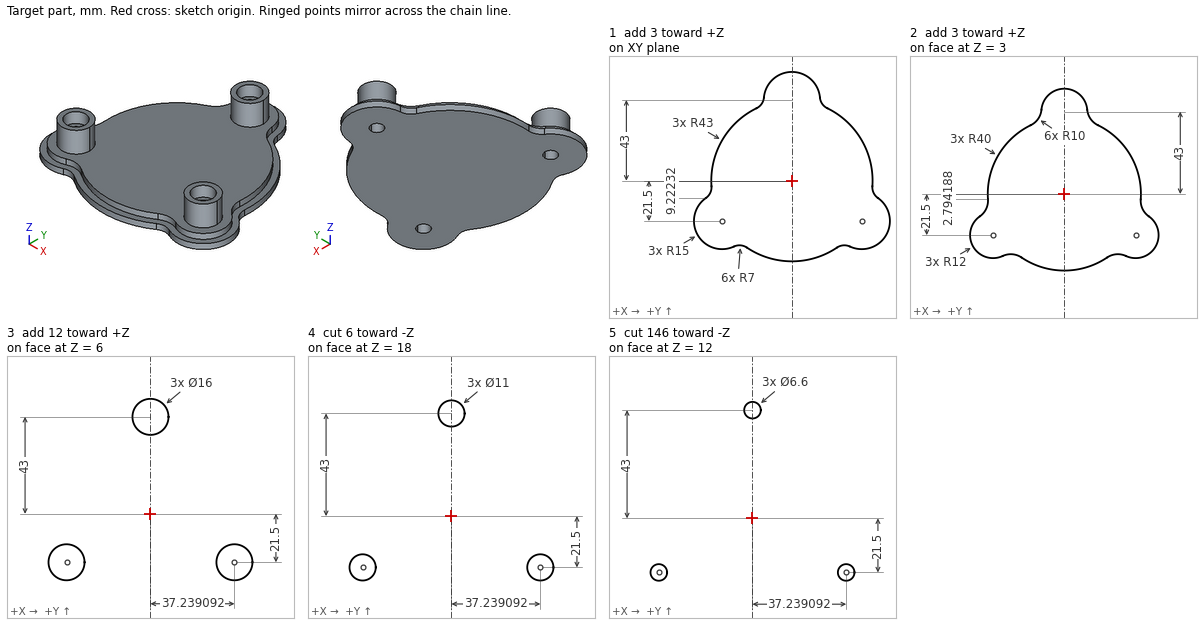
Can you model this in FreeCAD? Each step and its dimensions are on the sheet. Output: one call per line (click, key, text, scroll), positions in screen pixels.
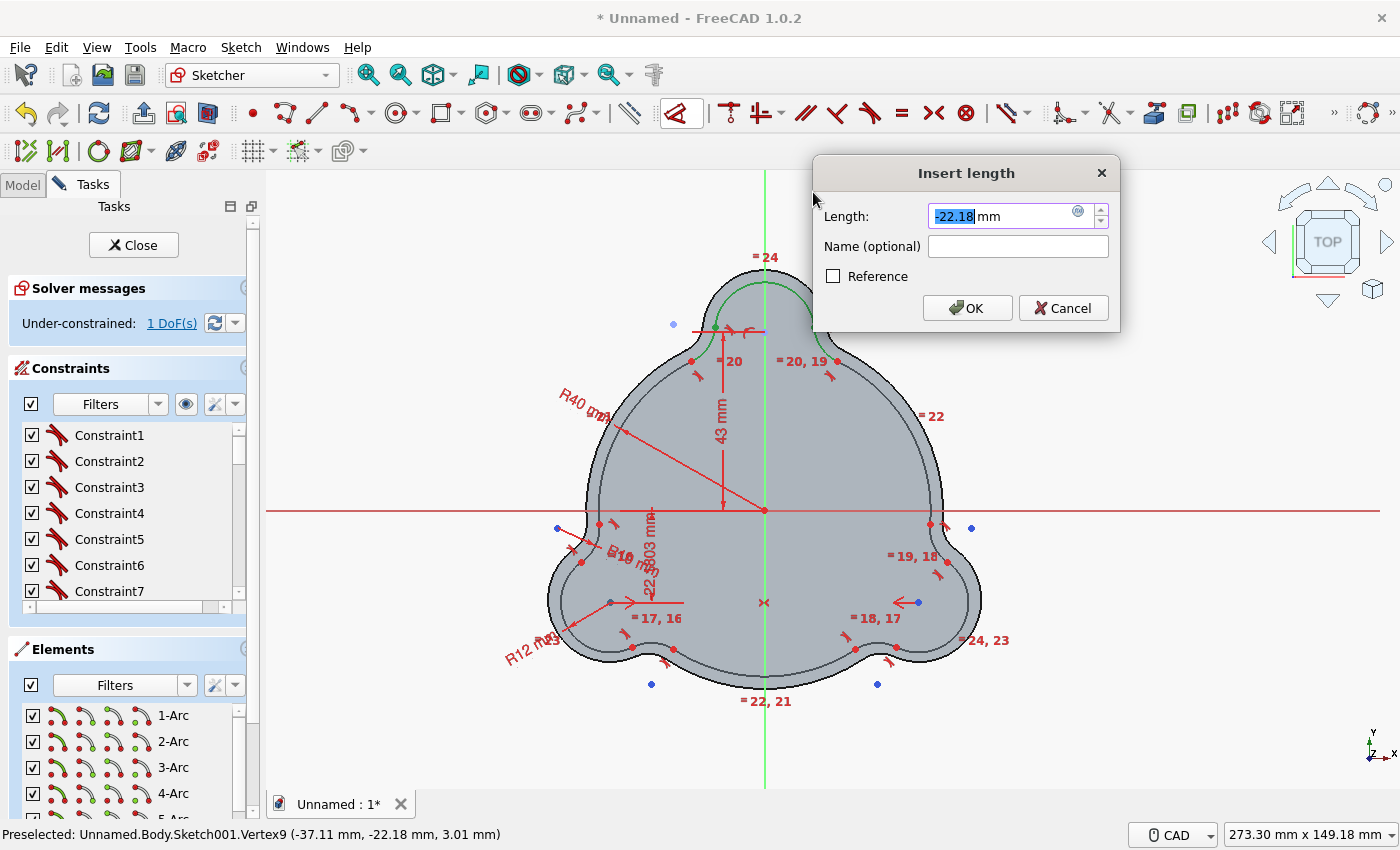
text(-21.5)
key(Return)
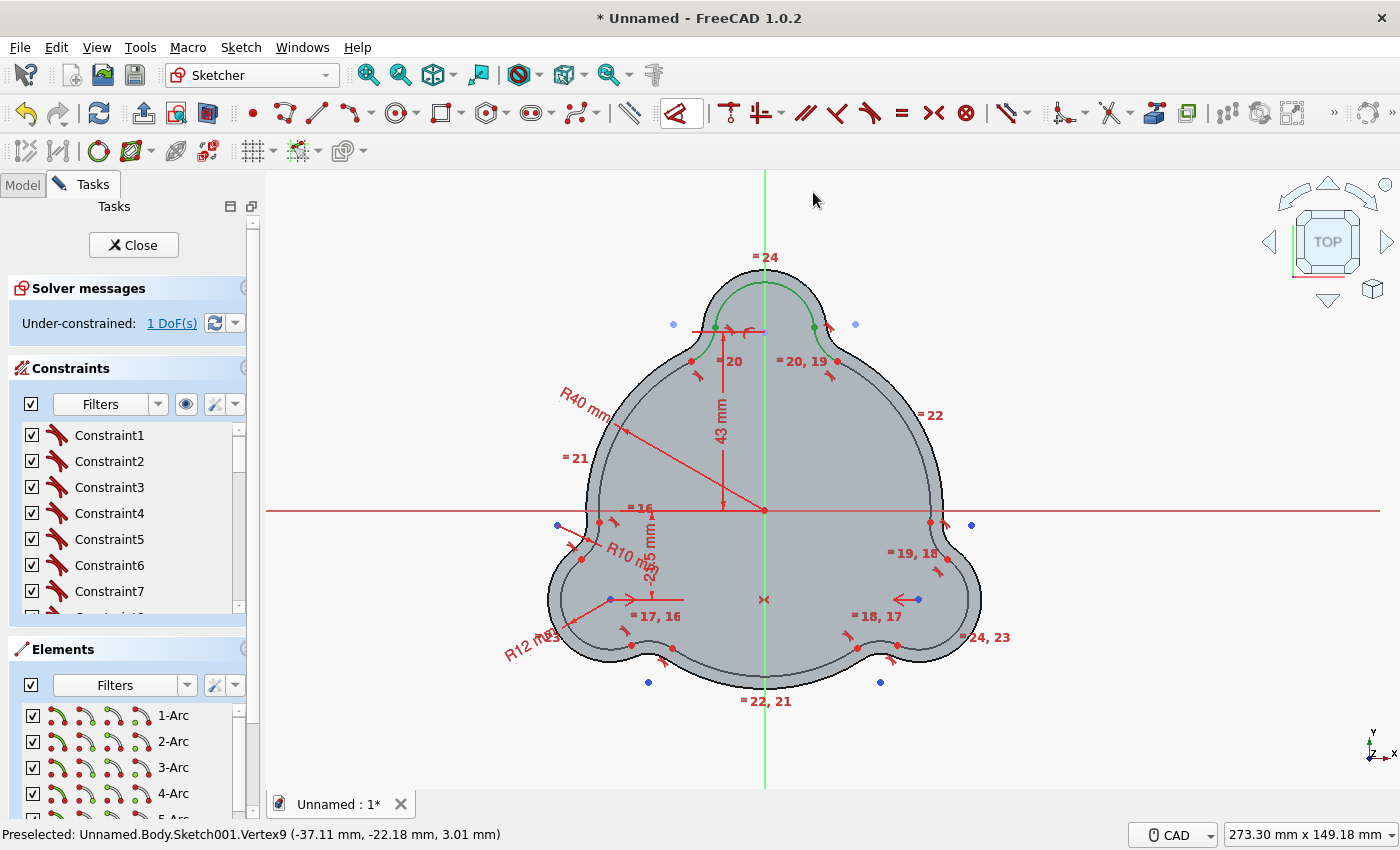
scroll(599, 522, up, 7)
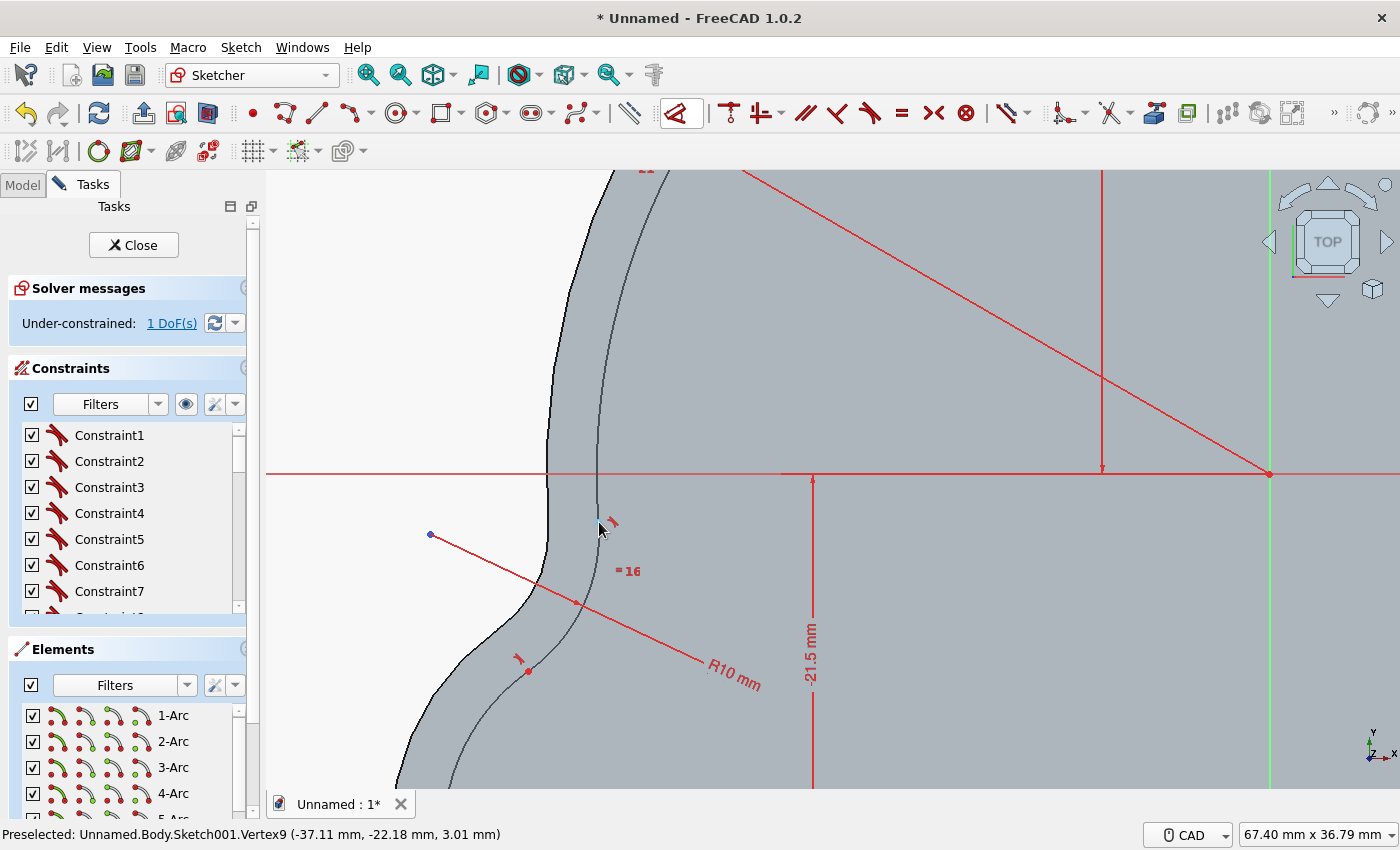
click(599, 522)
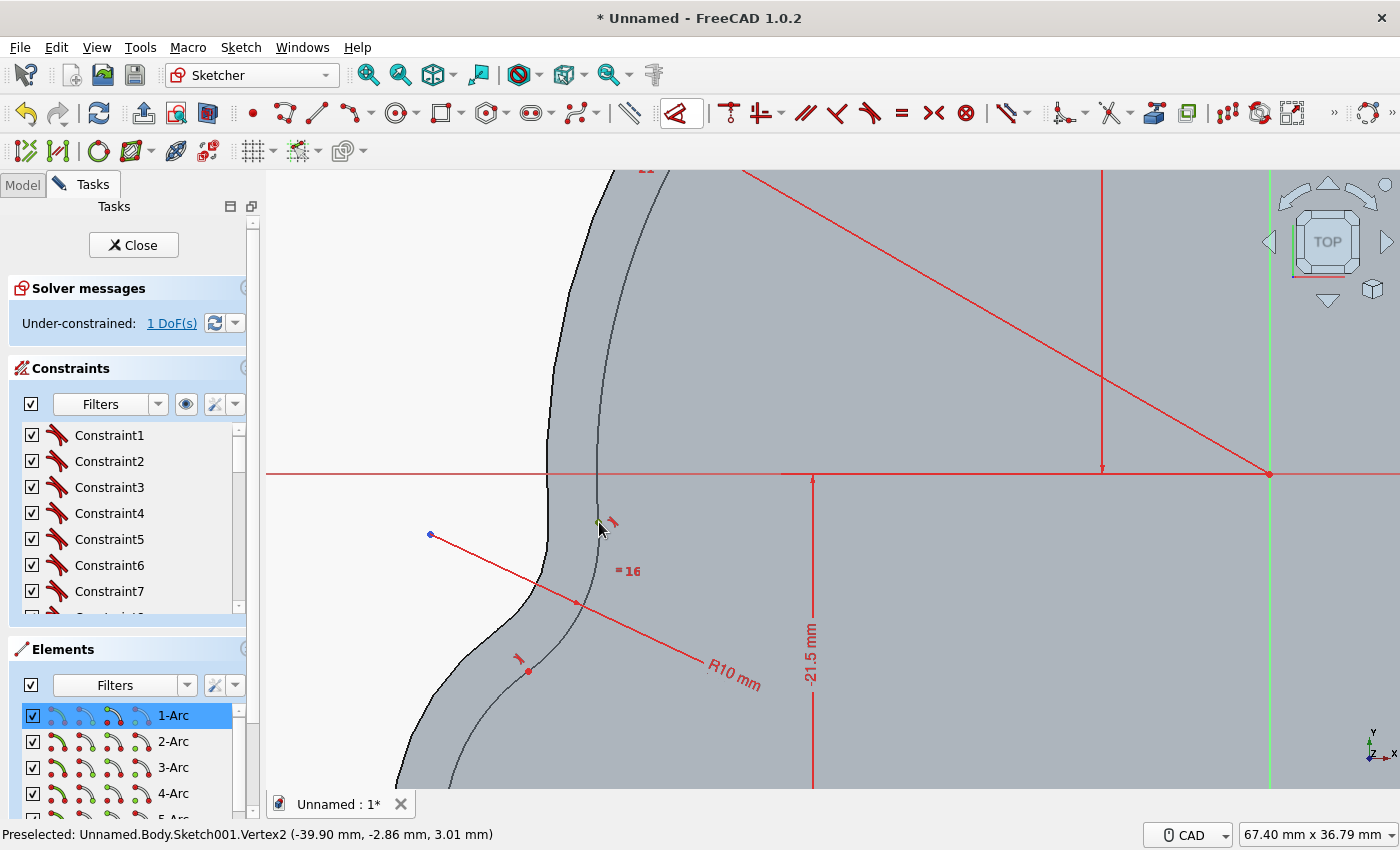
click(698, 114)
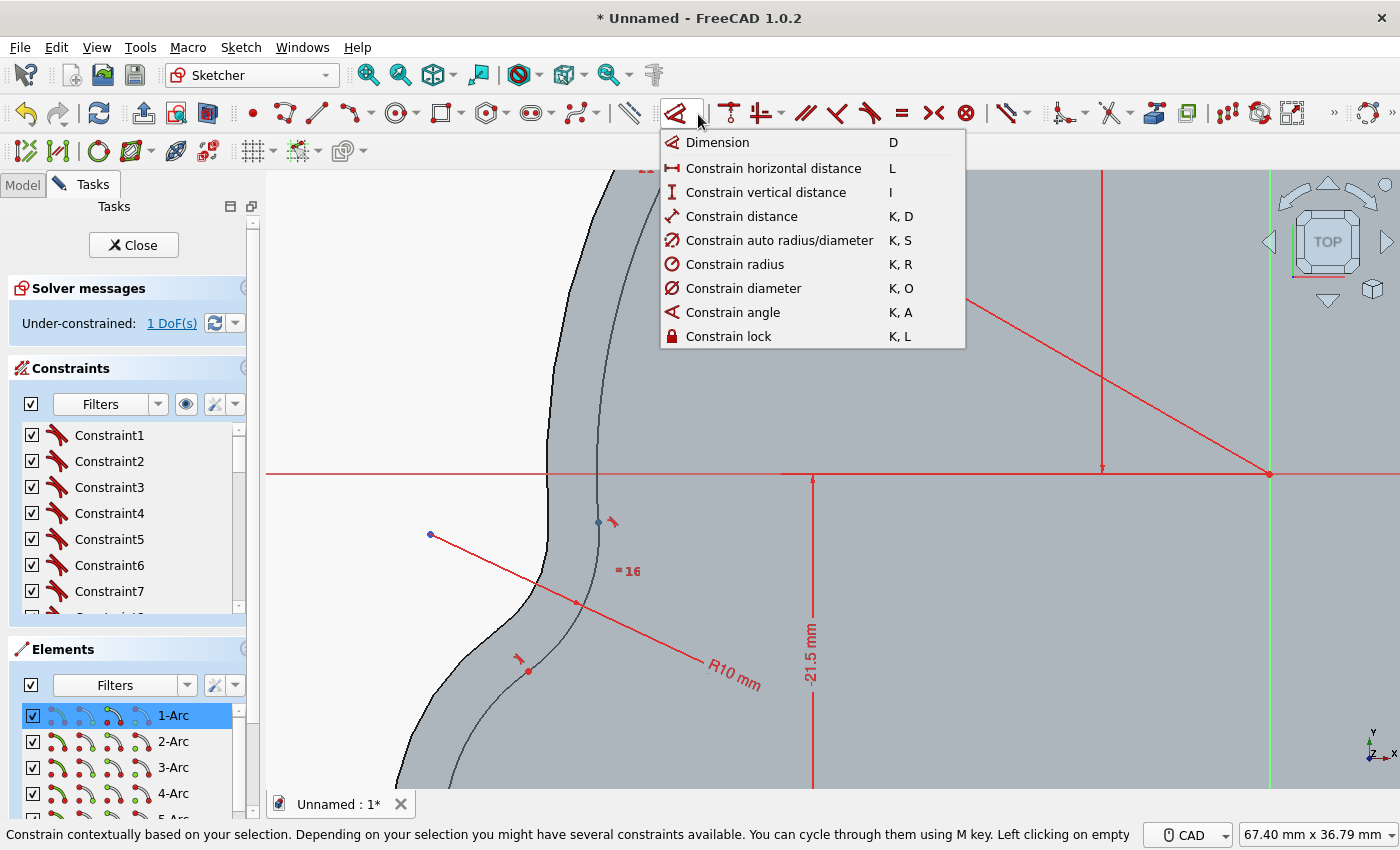
click(813, 192)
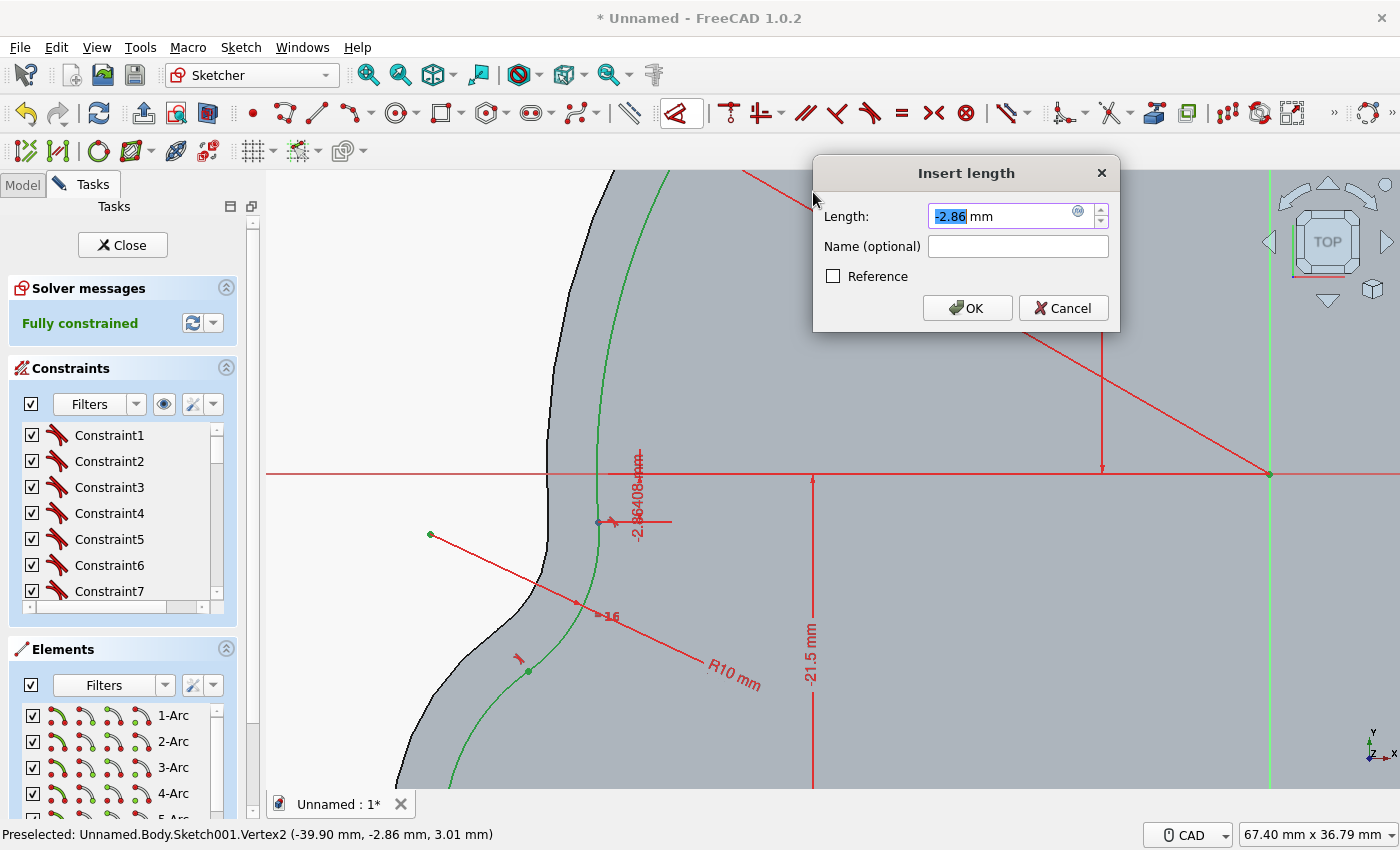
text(-2.794188)
key(Return)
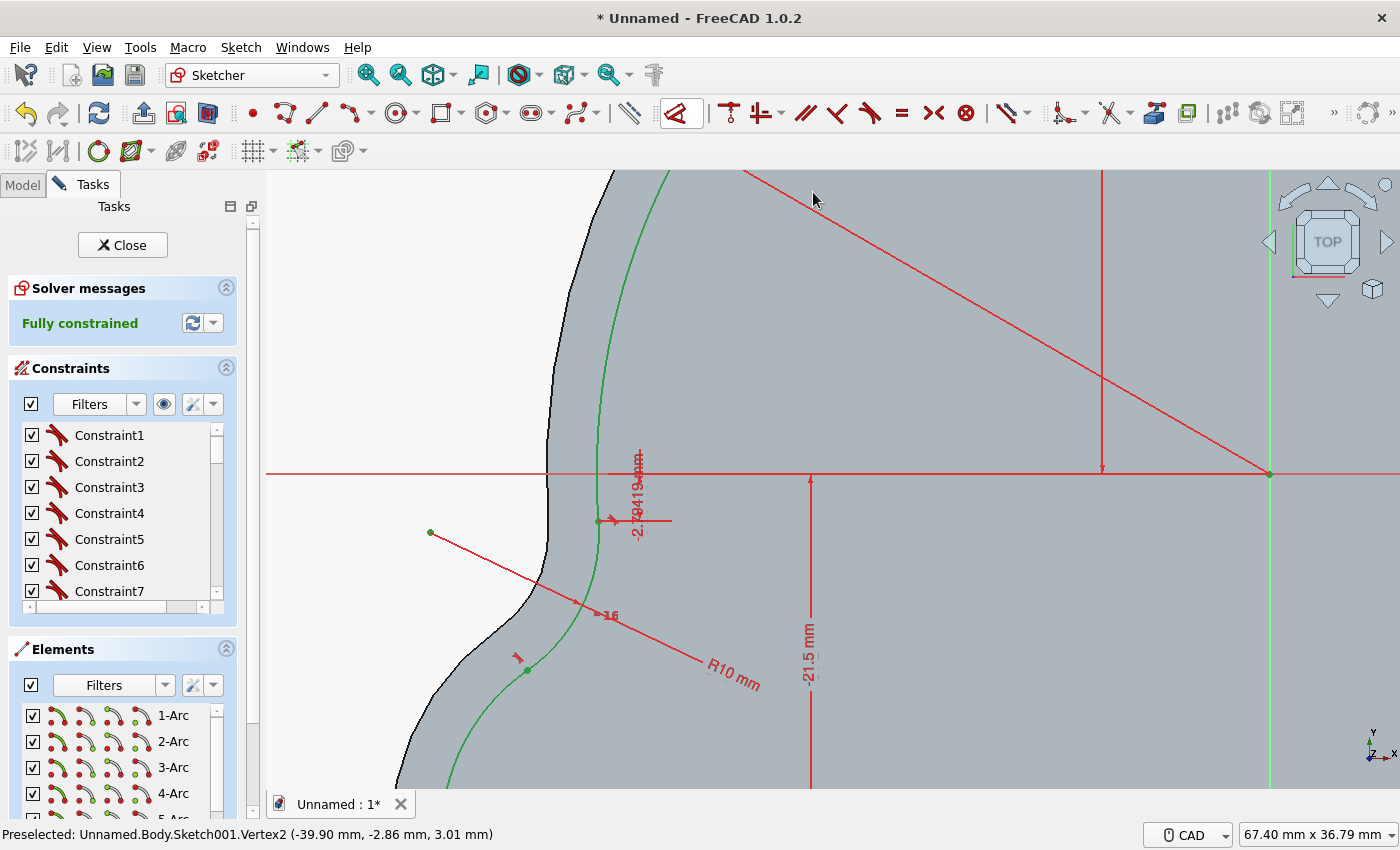
click(123, 245)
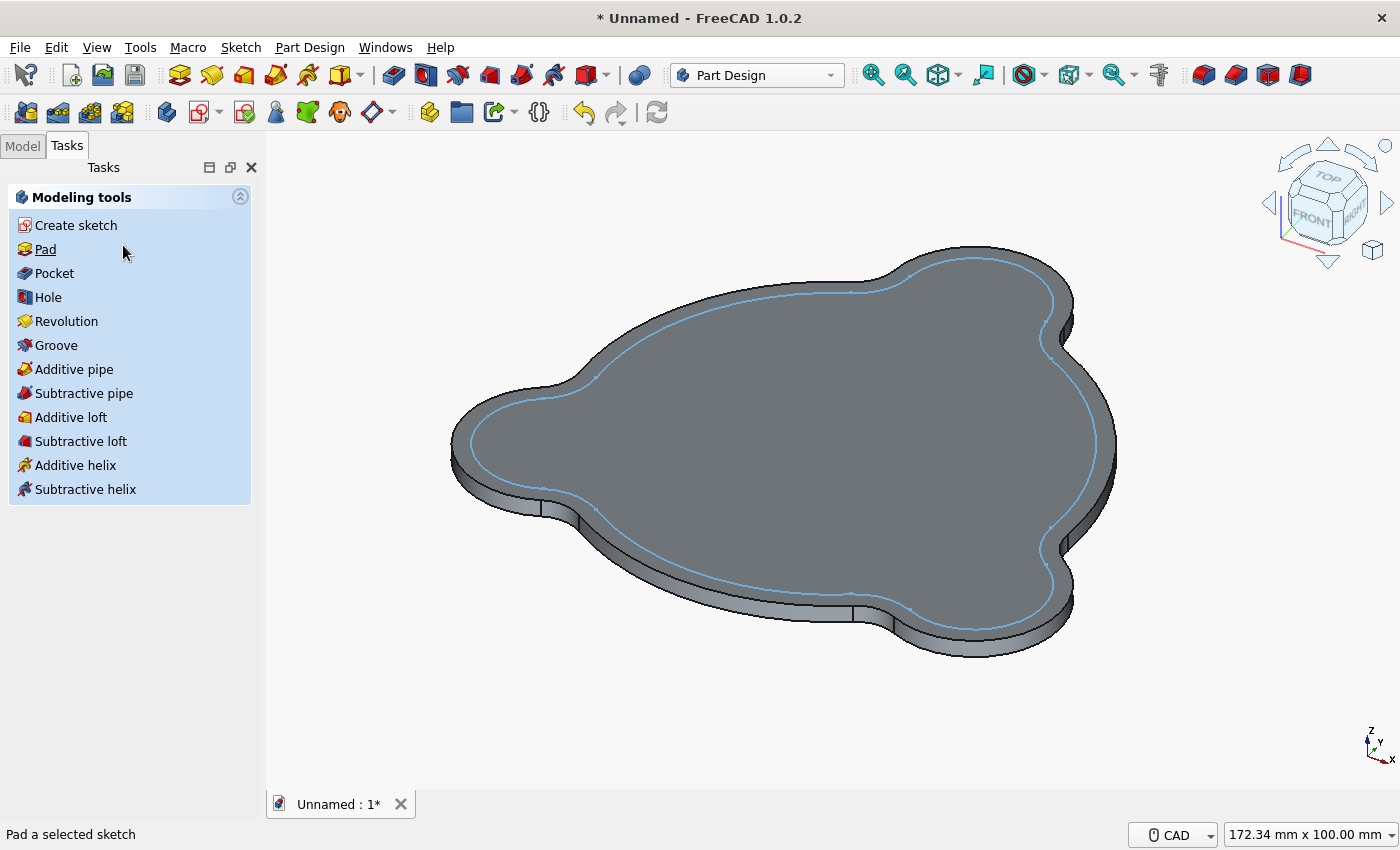
click(180, 76)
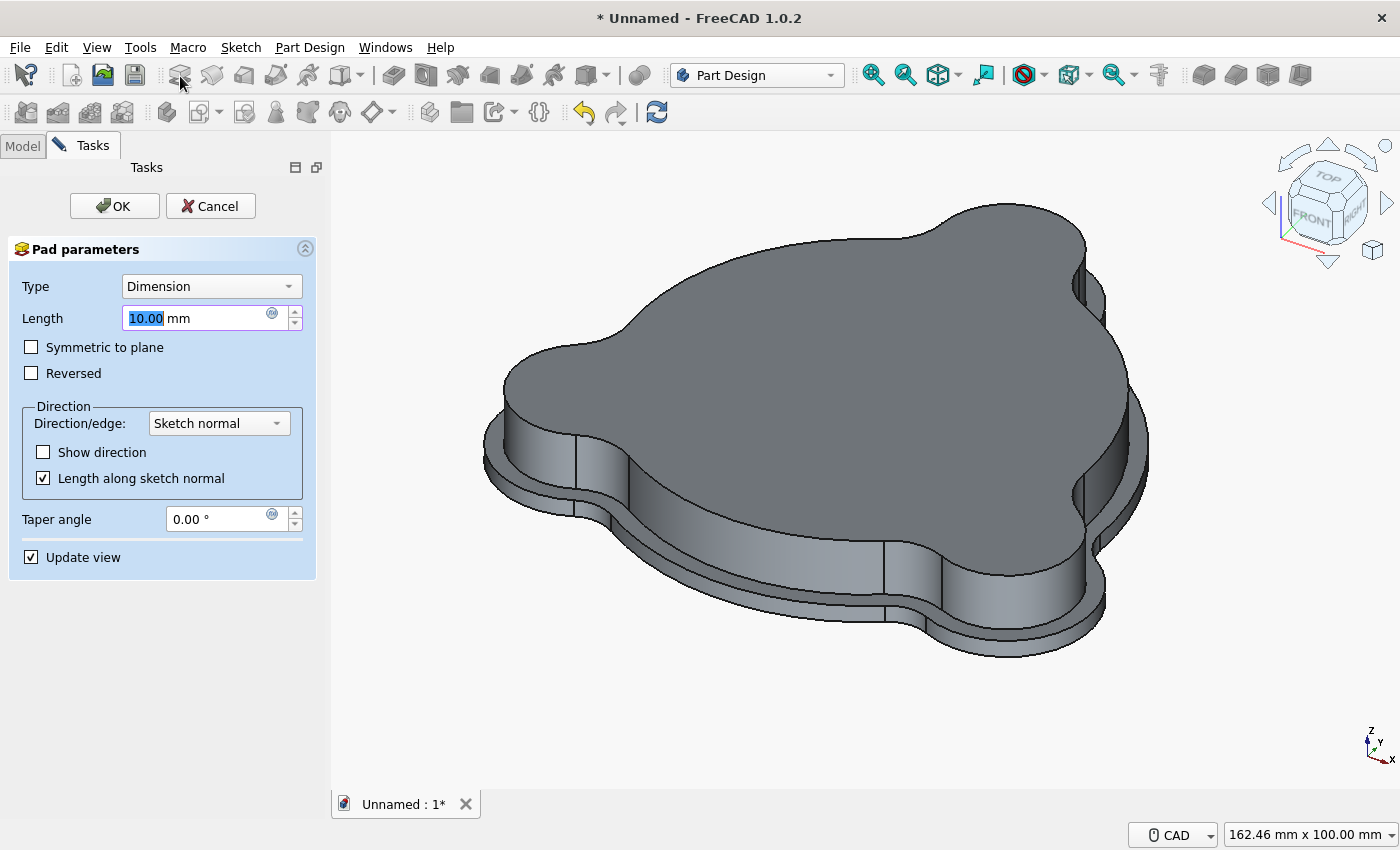
text(3)
key(Tab)